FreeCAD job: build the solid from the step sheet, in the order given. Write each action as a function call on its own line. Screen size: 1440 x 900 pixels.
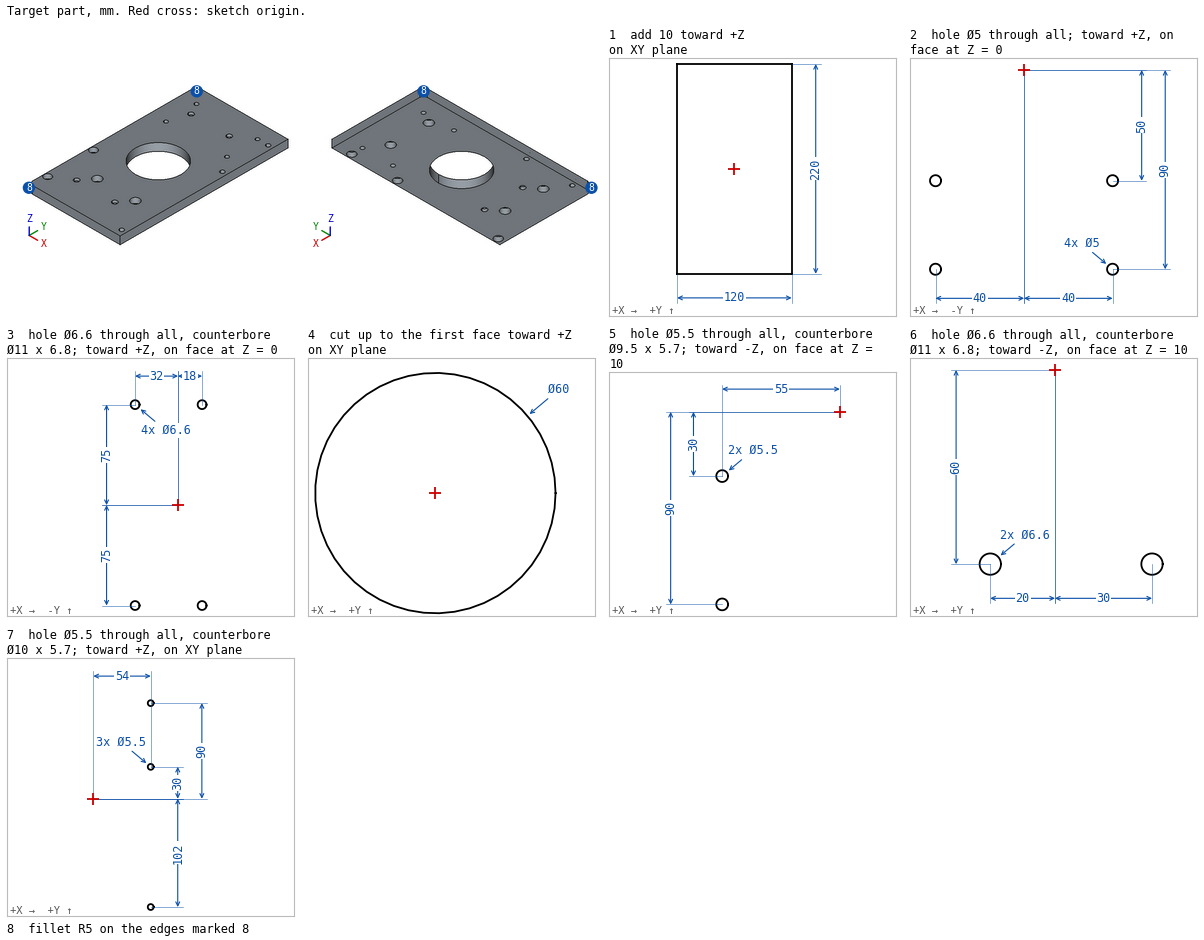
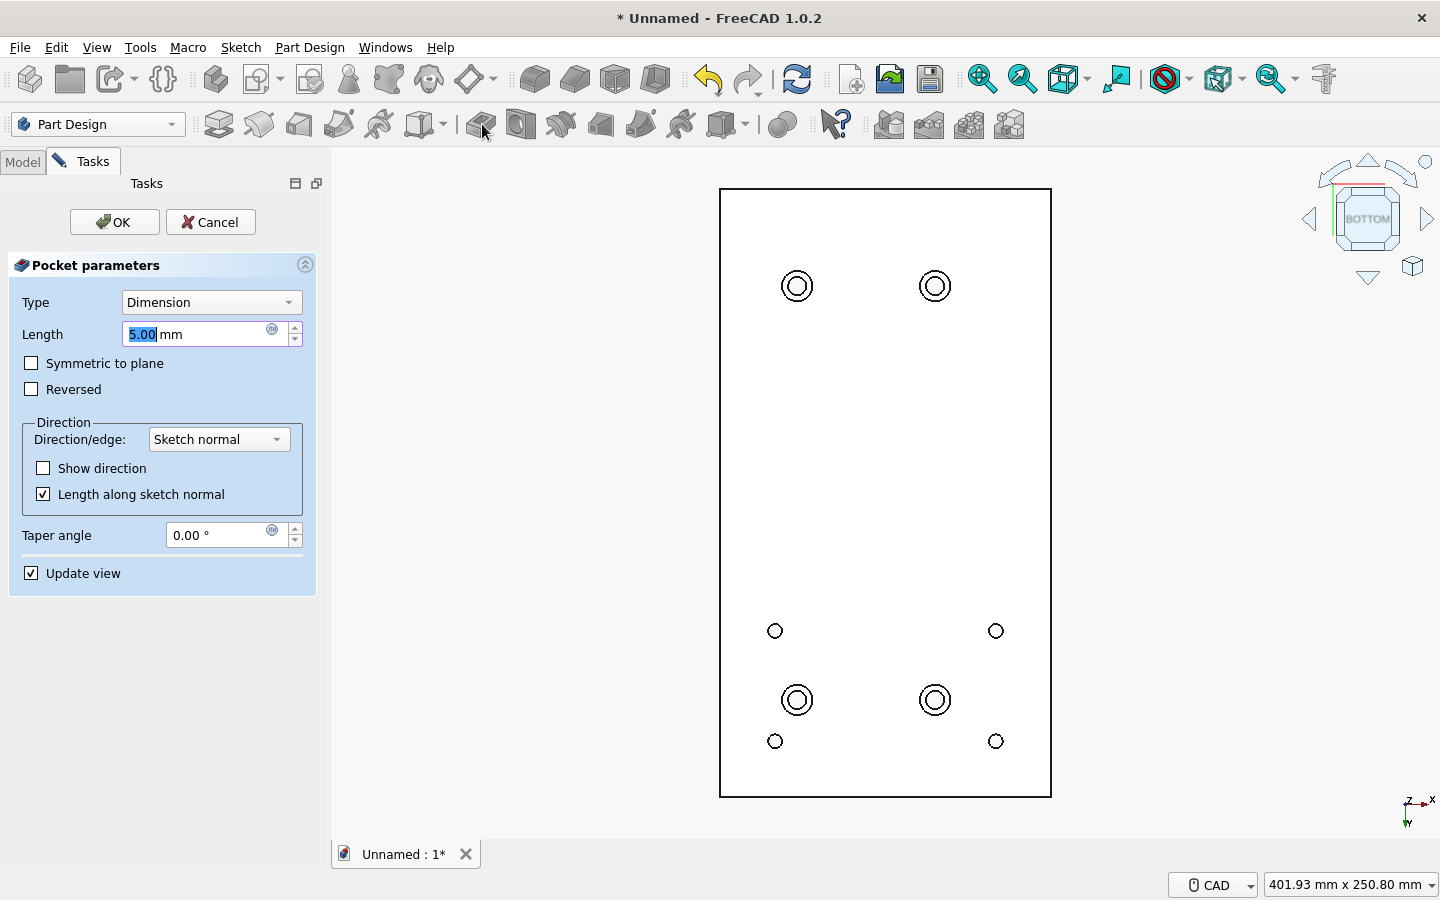
click(212, 302)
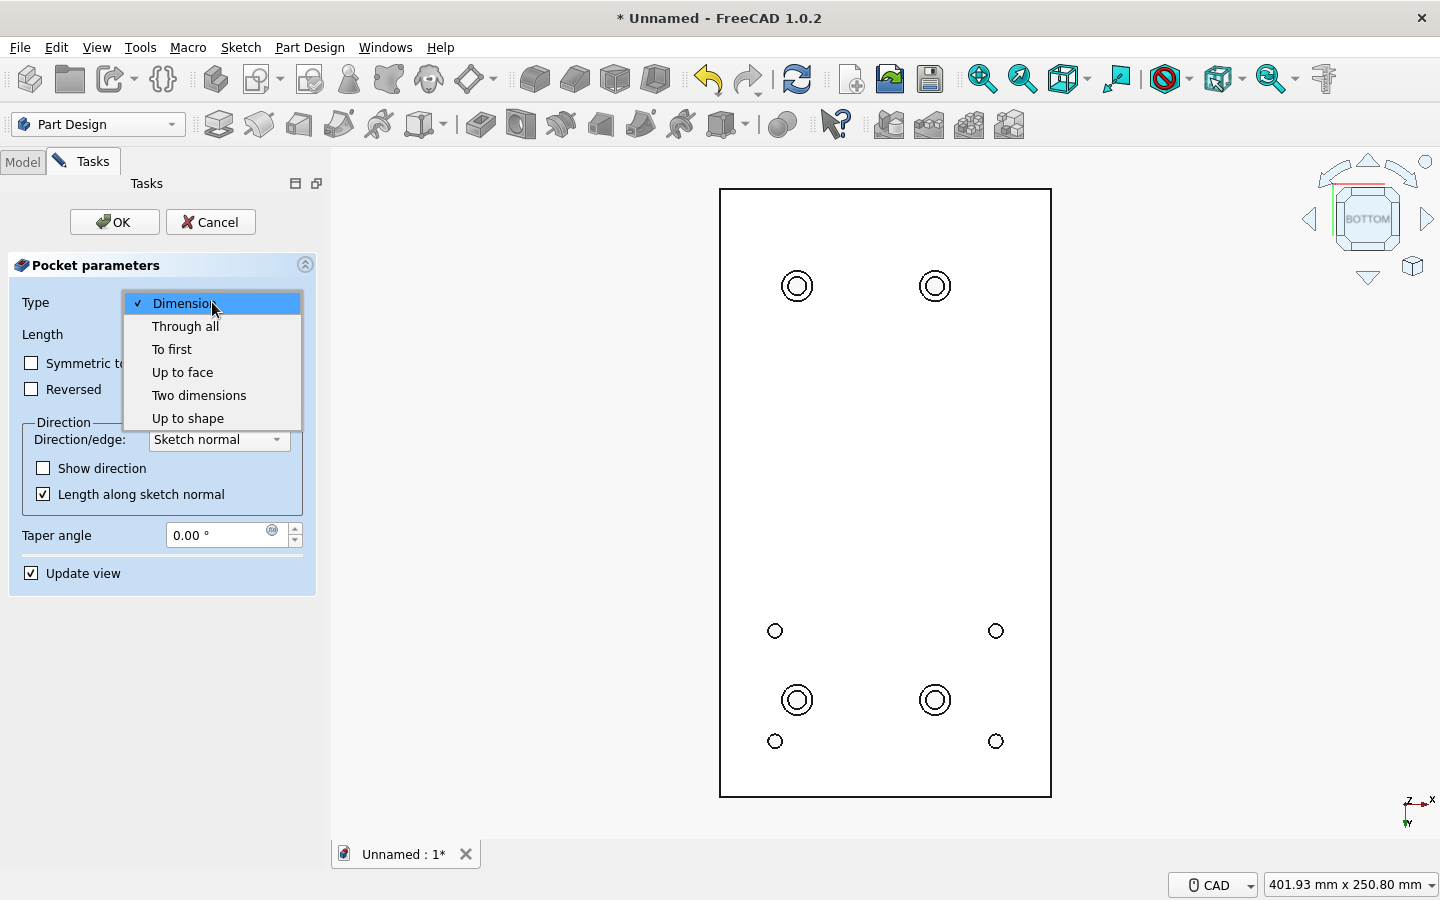
click(212, 350)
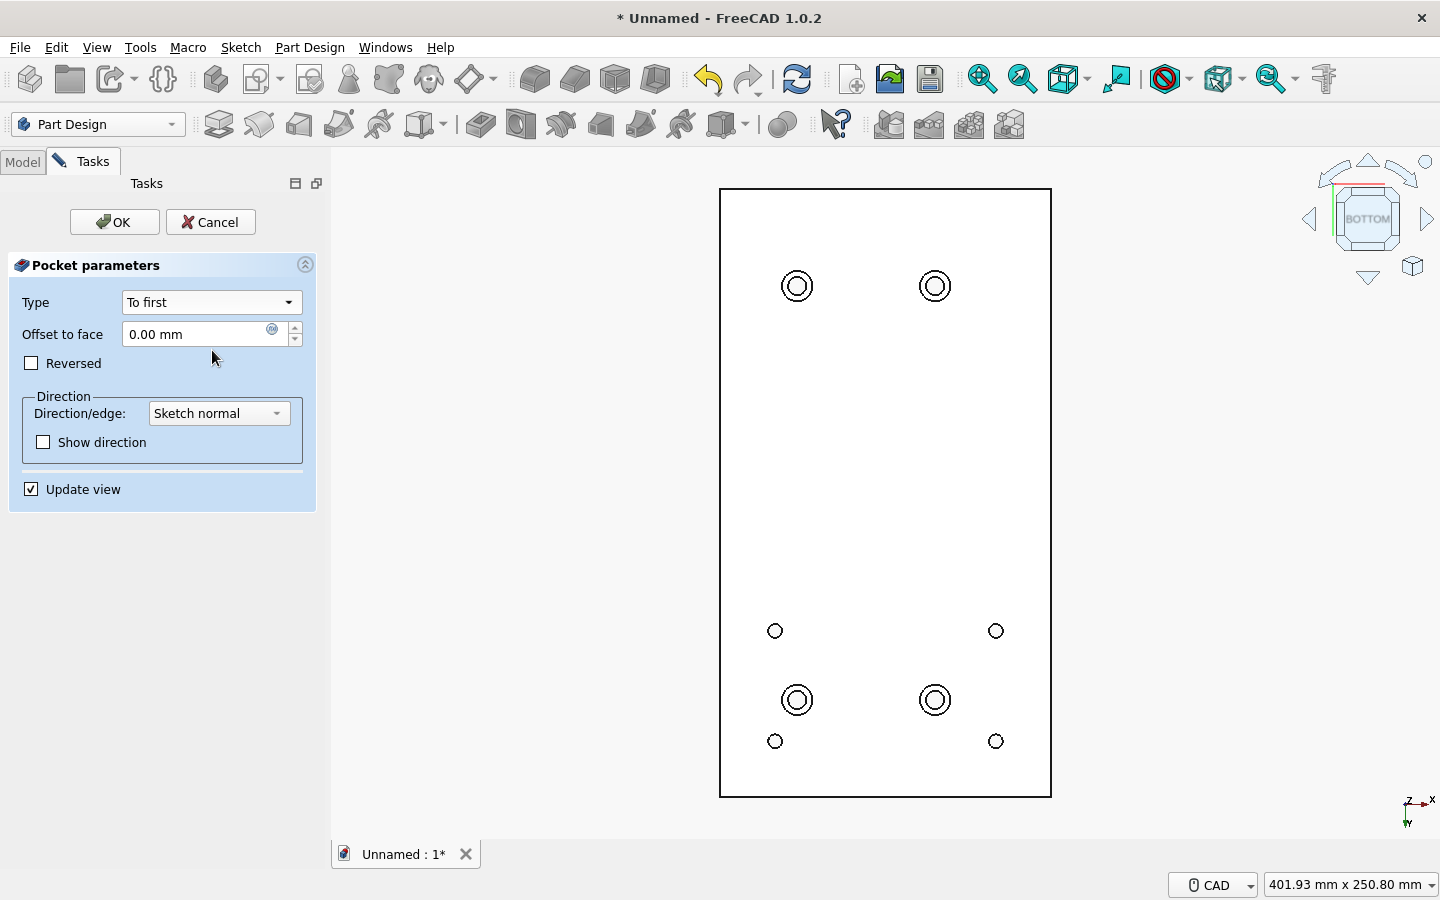
click(30, 363)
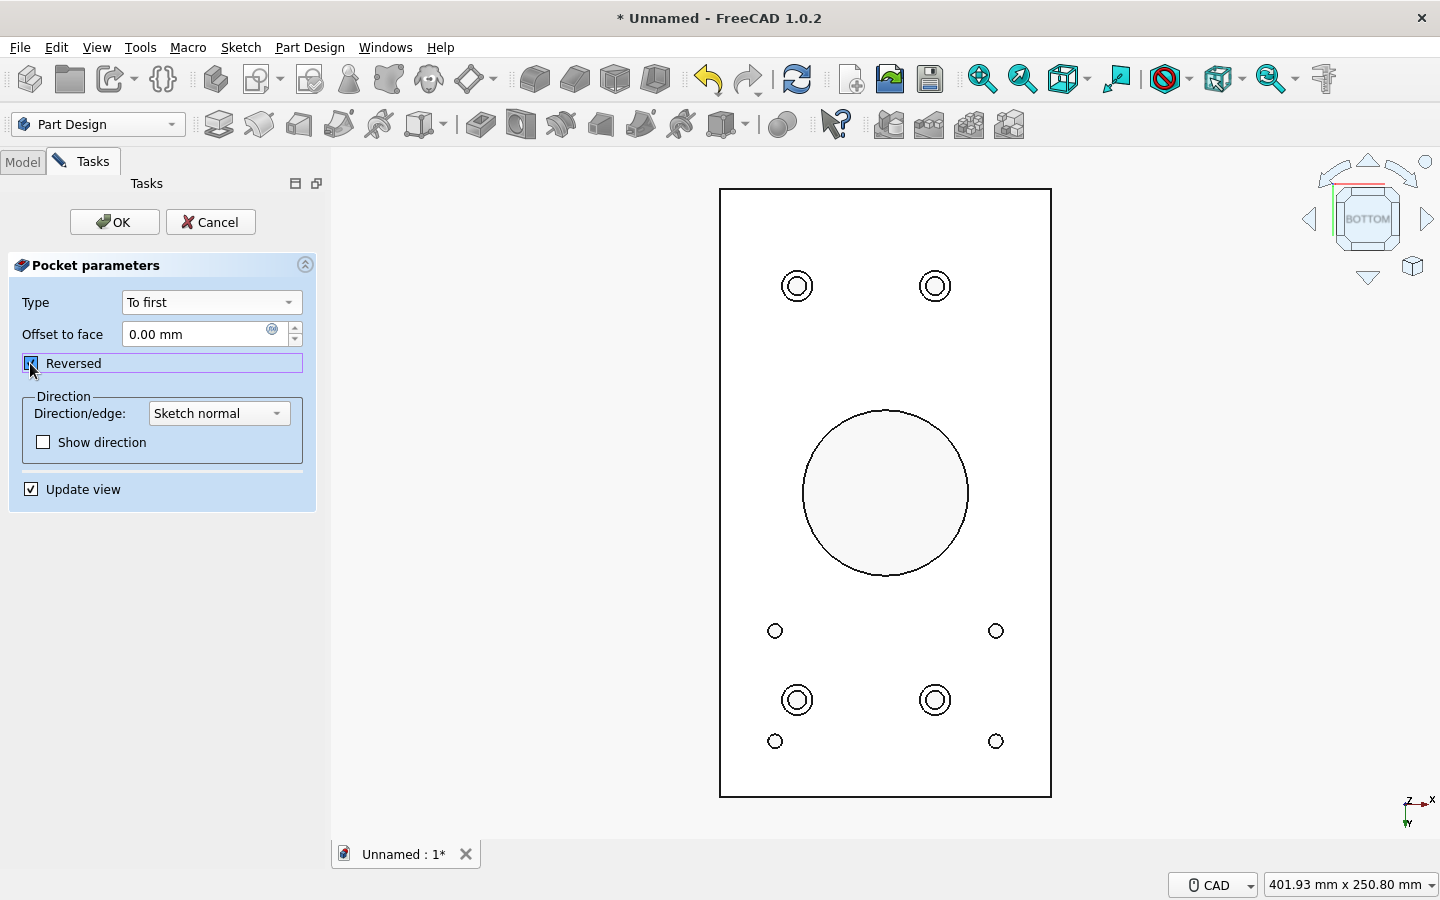
click(115, 222)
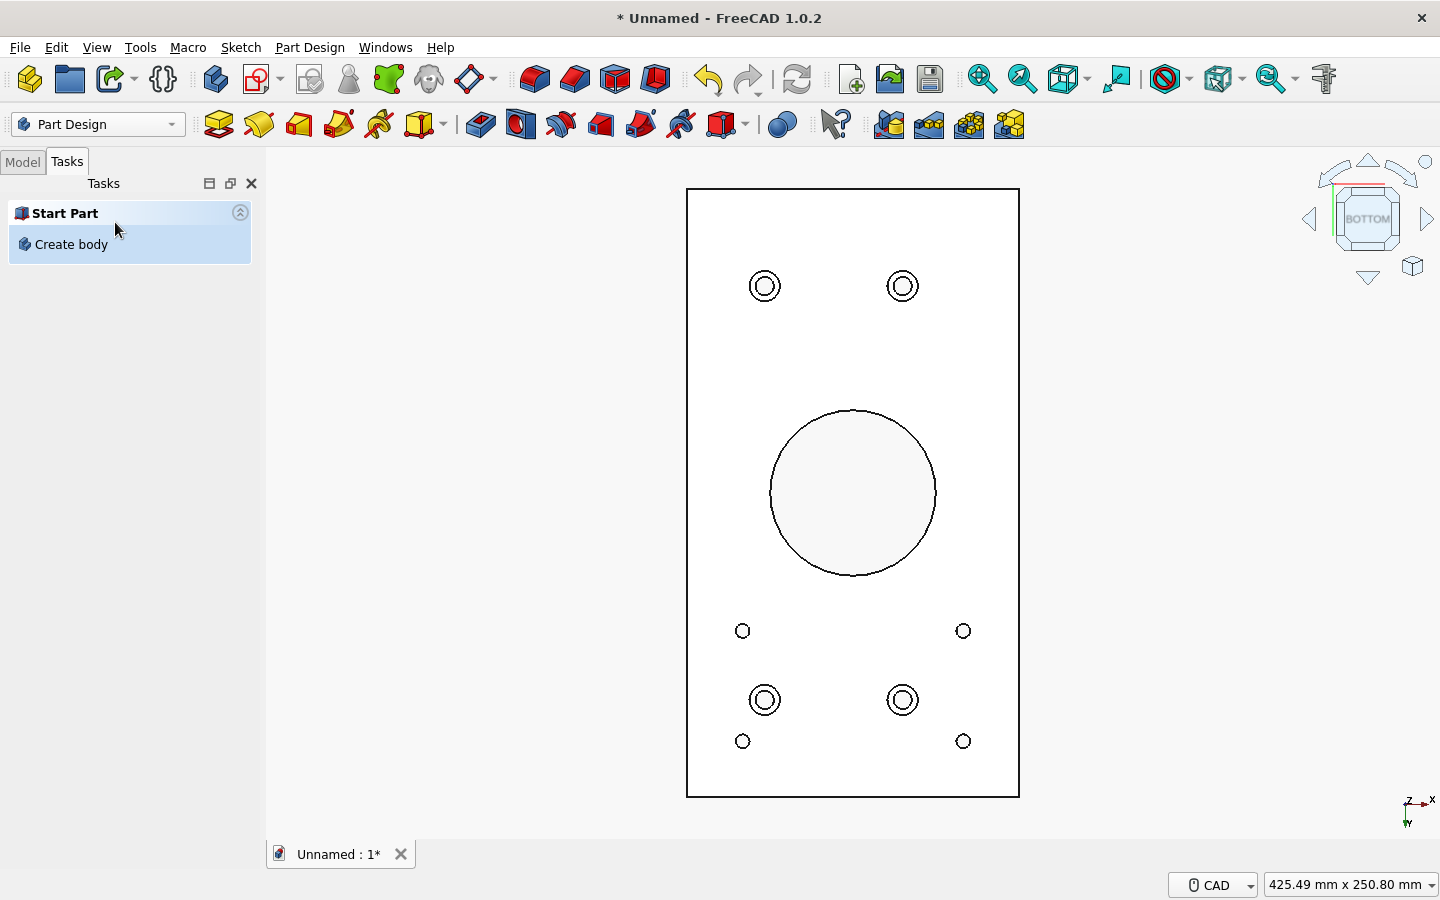
key(0)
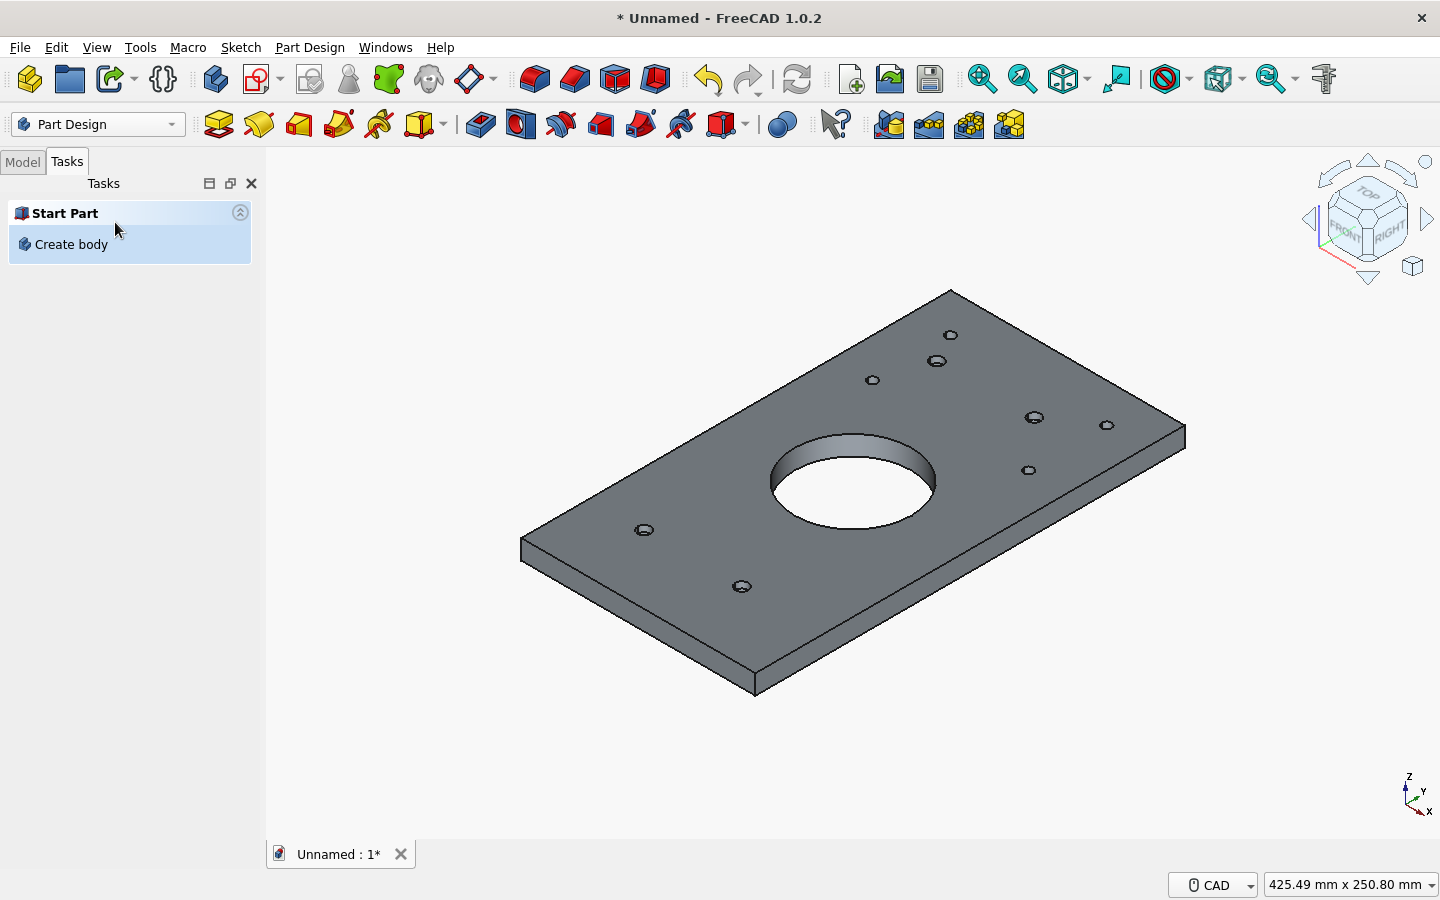
click(730, 552)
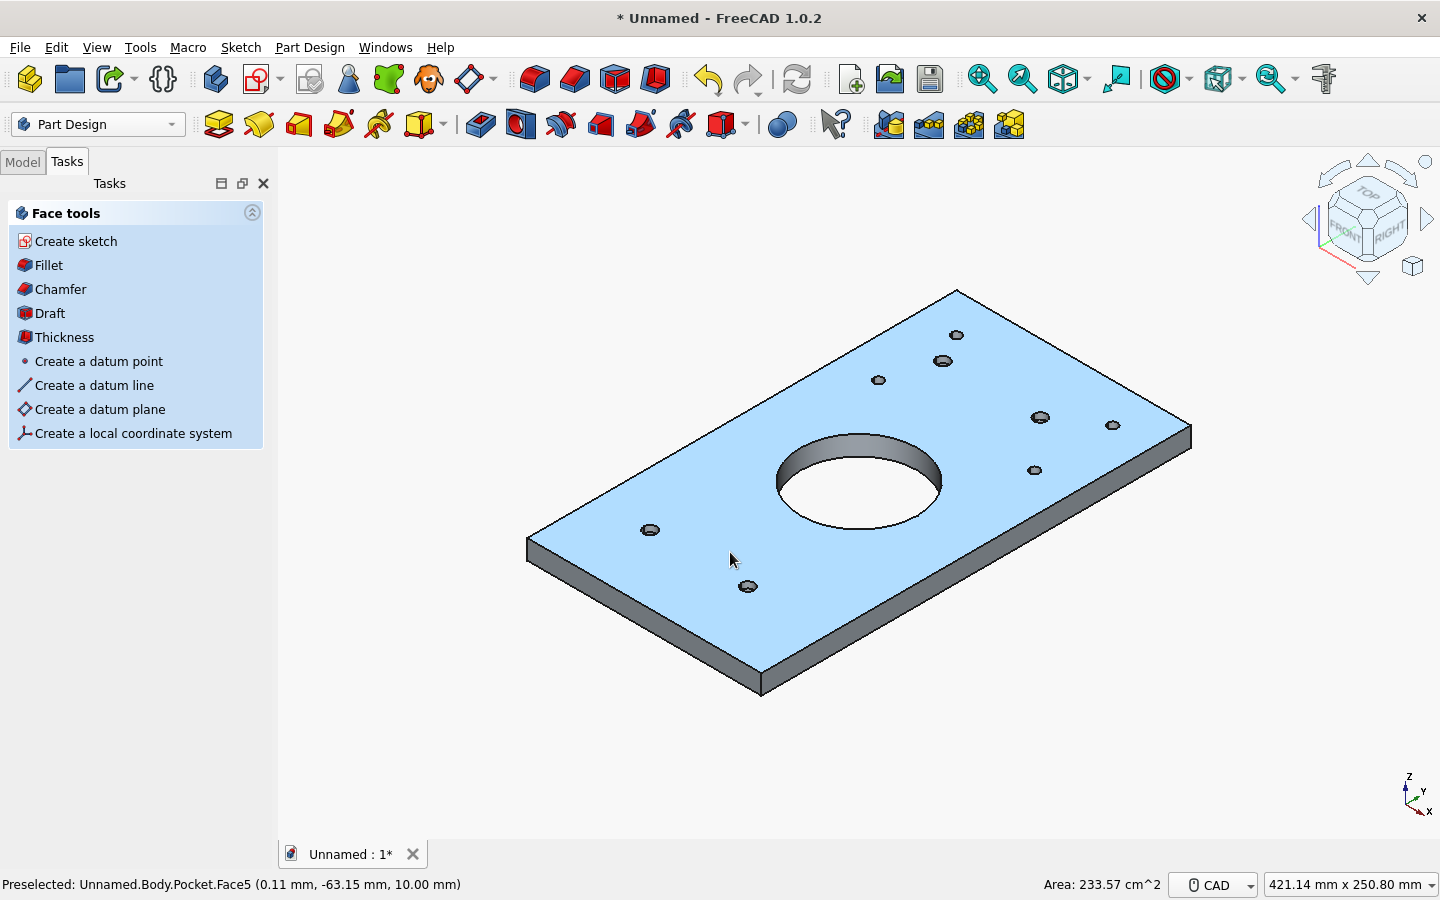
click(256, 80)